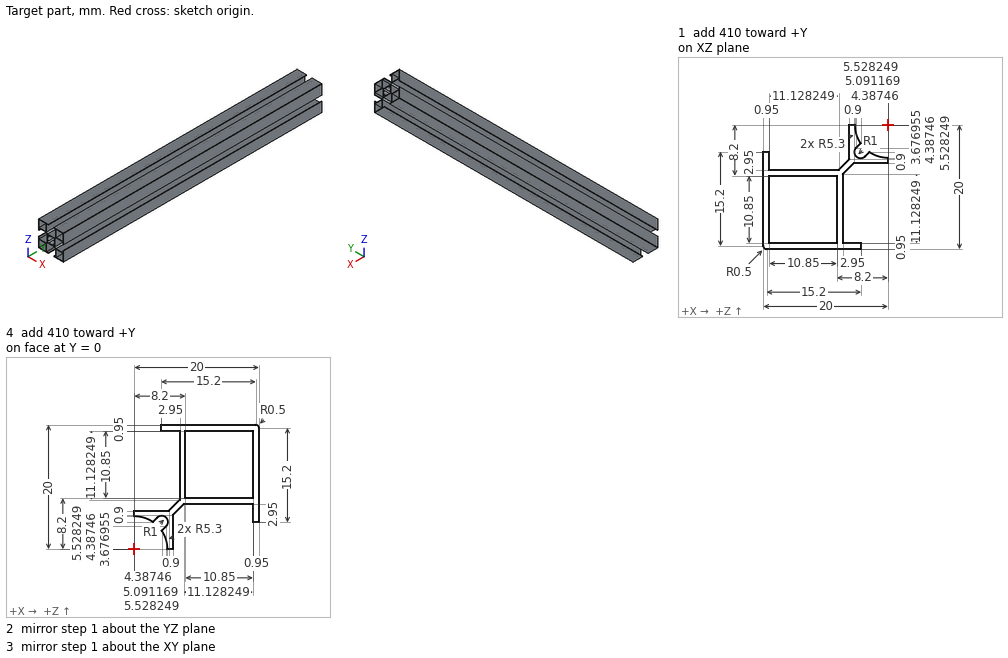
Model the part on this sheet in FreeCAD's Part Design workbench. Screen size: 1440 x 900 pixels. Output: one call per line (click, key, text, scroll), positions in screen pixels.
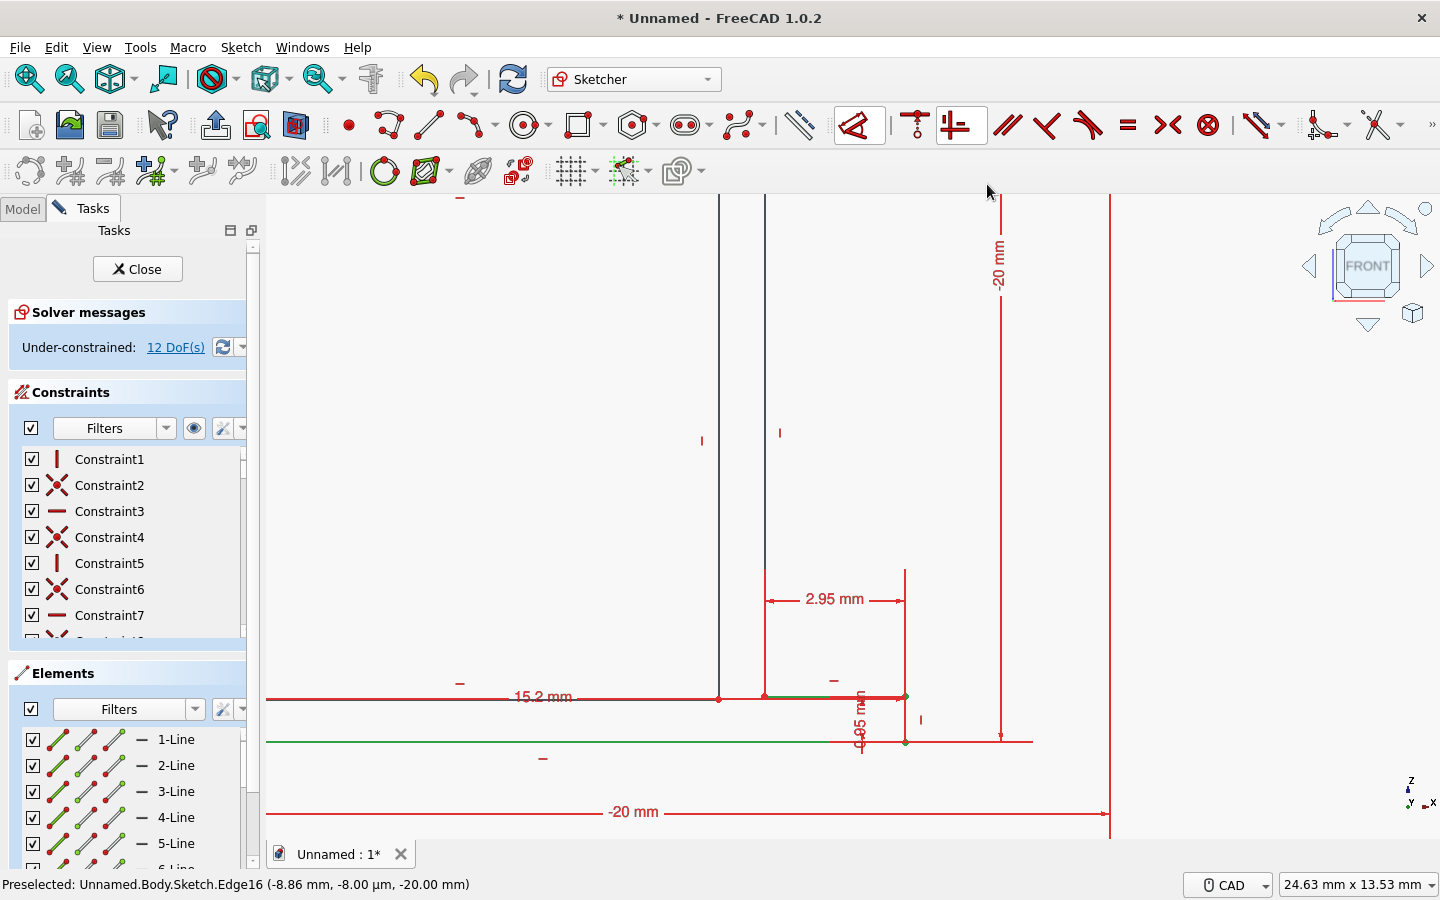
scroll(908, 721, down, 4)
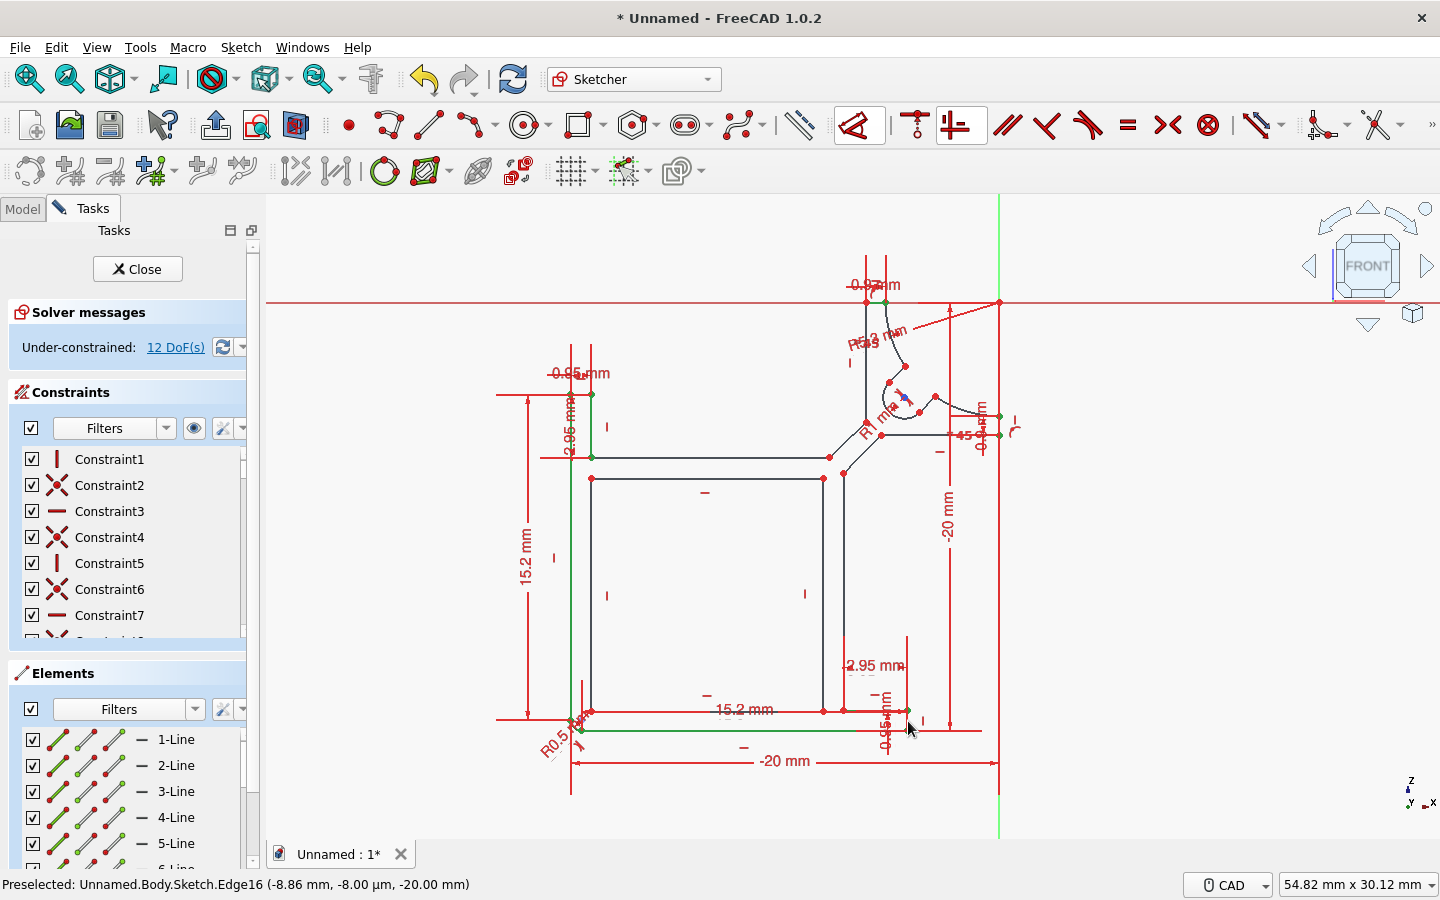
click(591, 479)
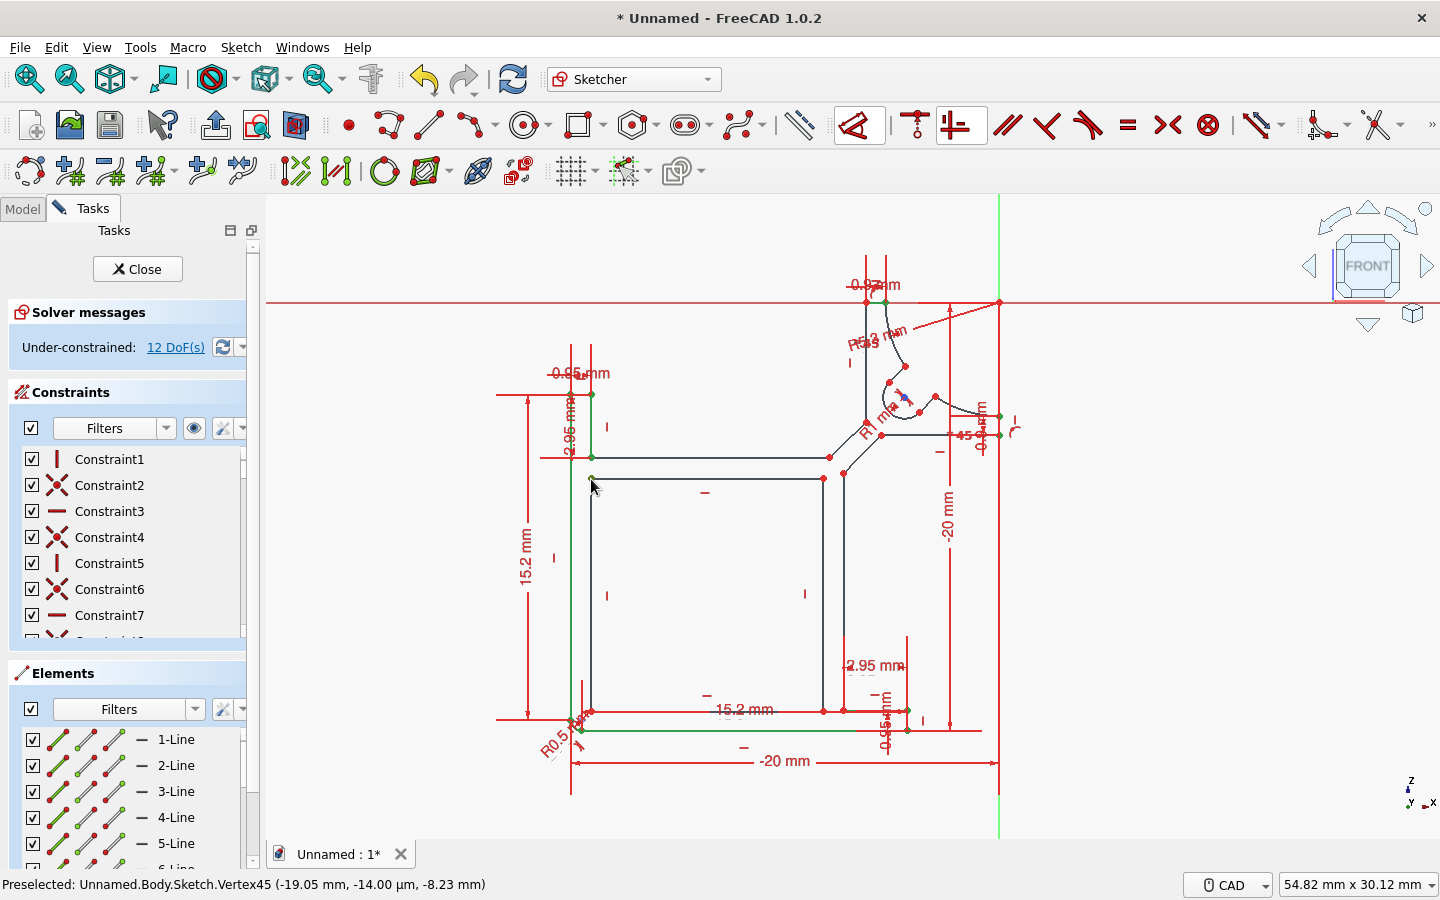
key(i)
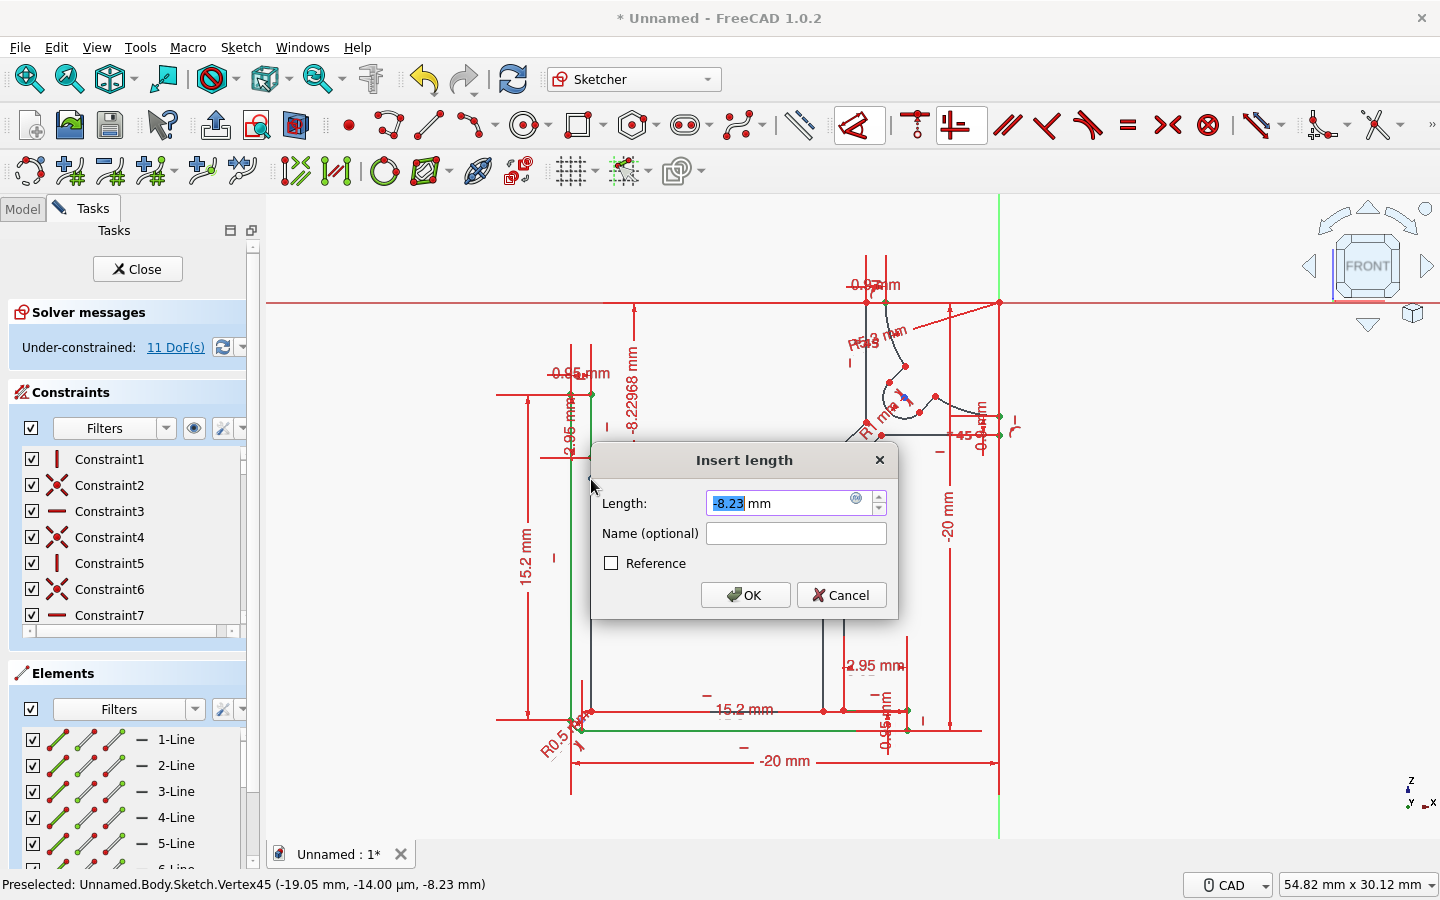
text(-8.2)
key(Return)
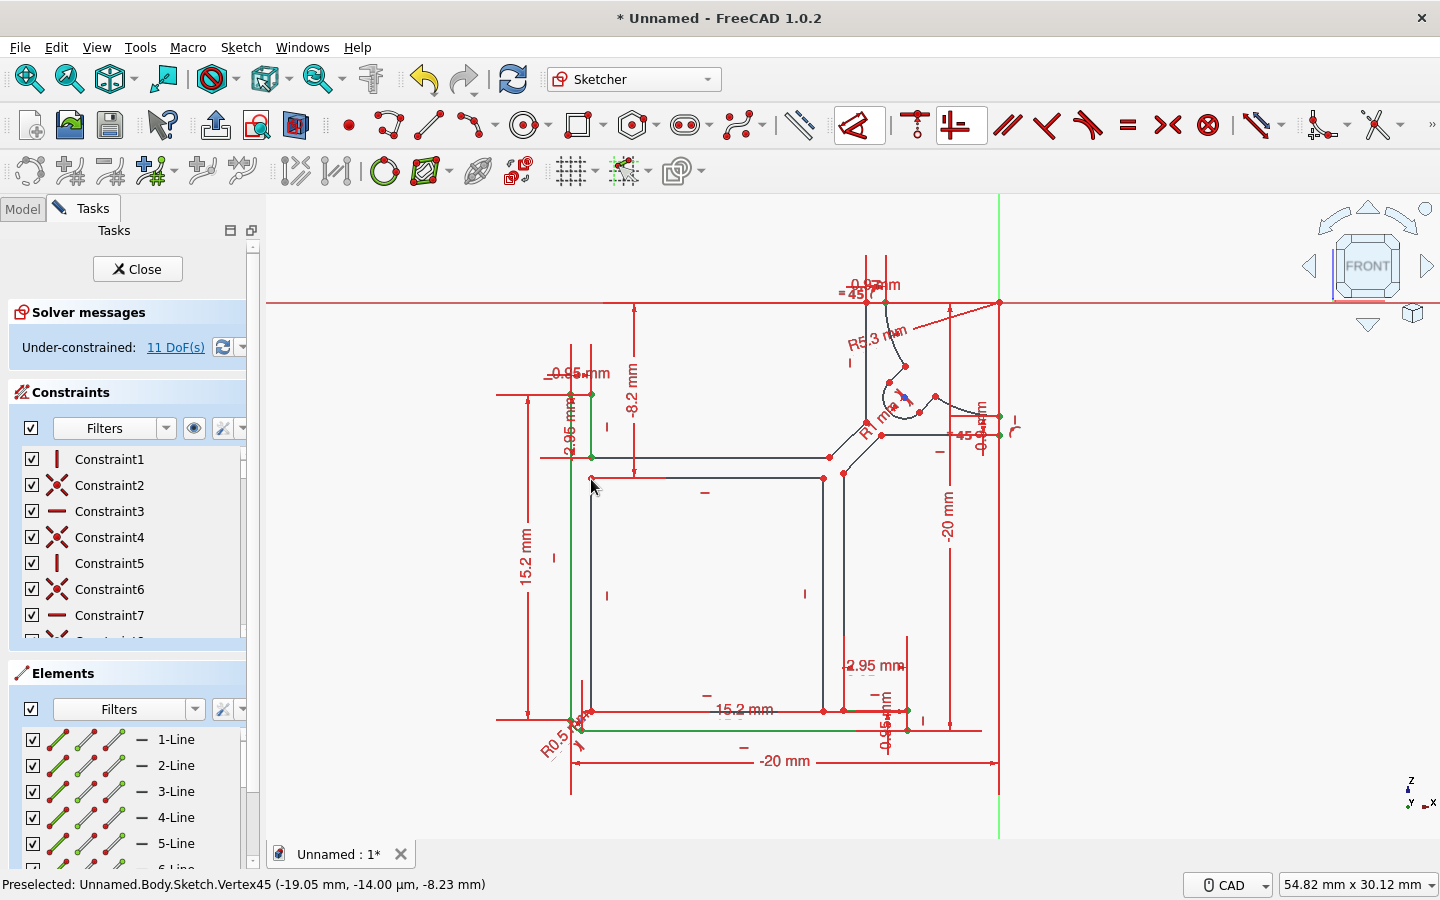
click(823, 712)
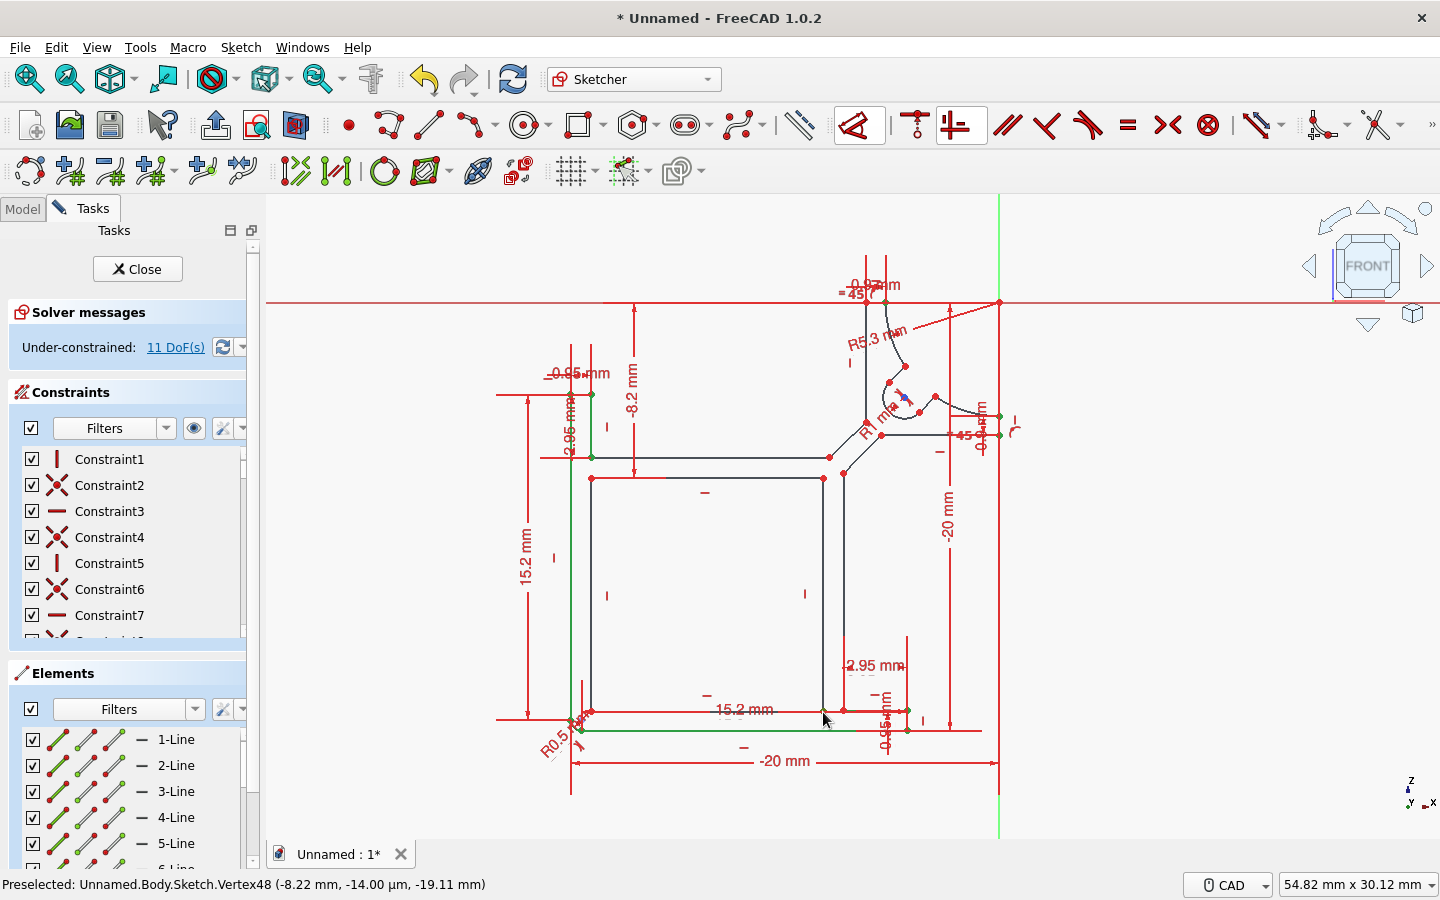
key(l)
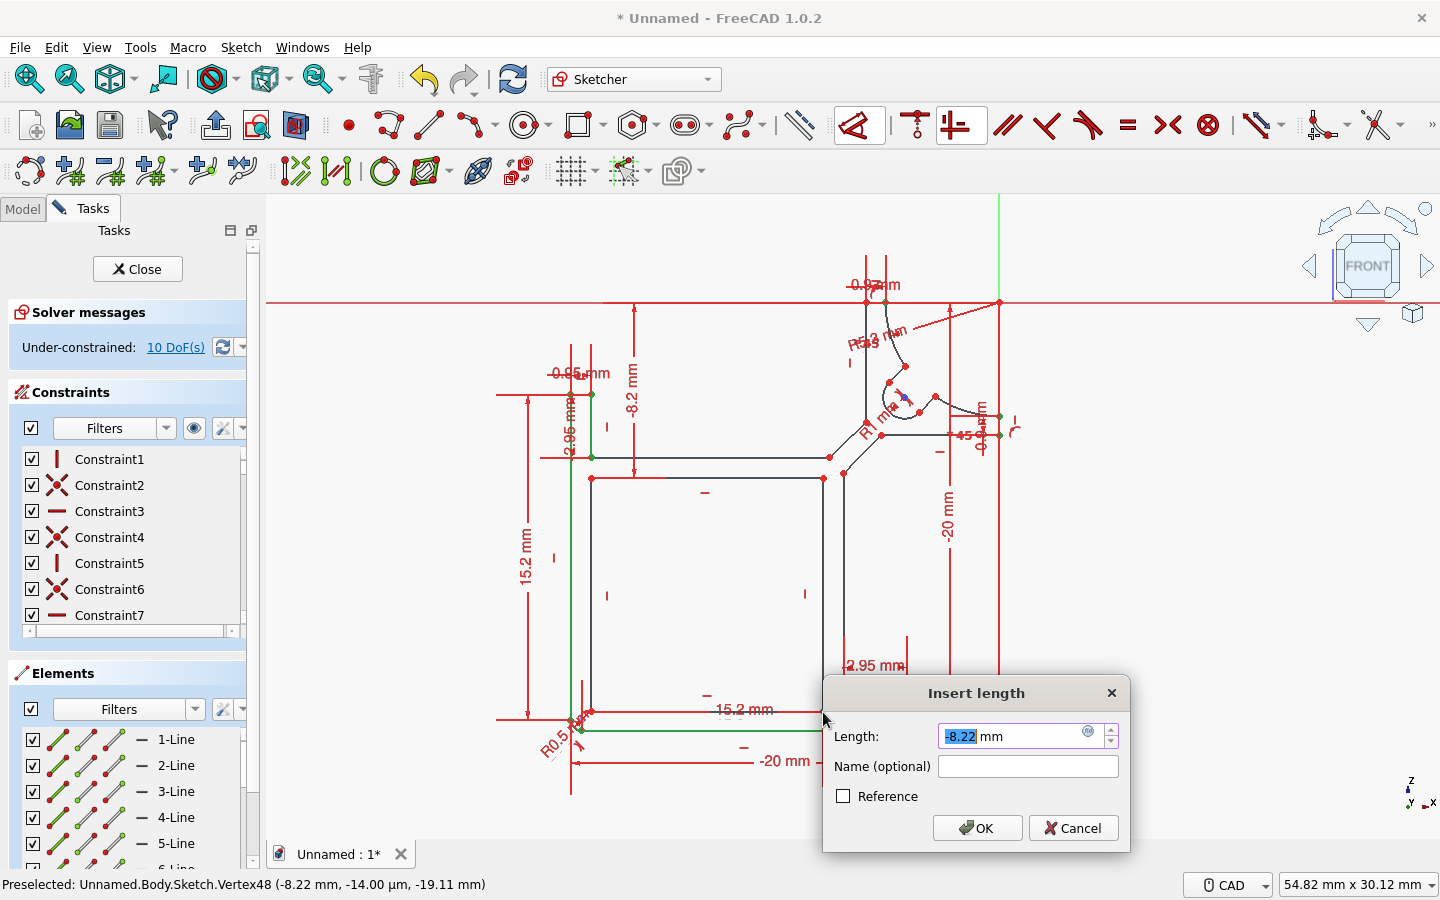
text(-8.2)
key(Return)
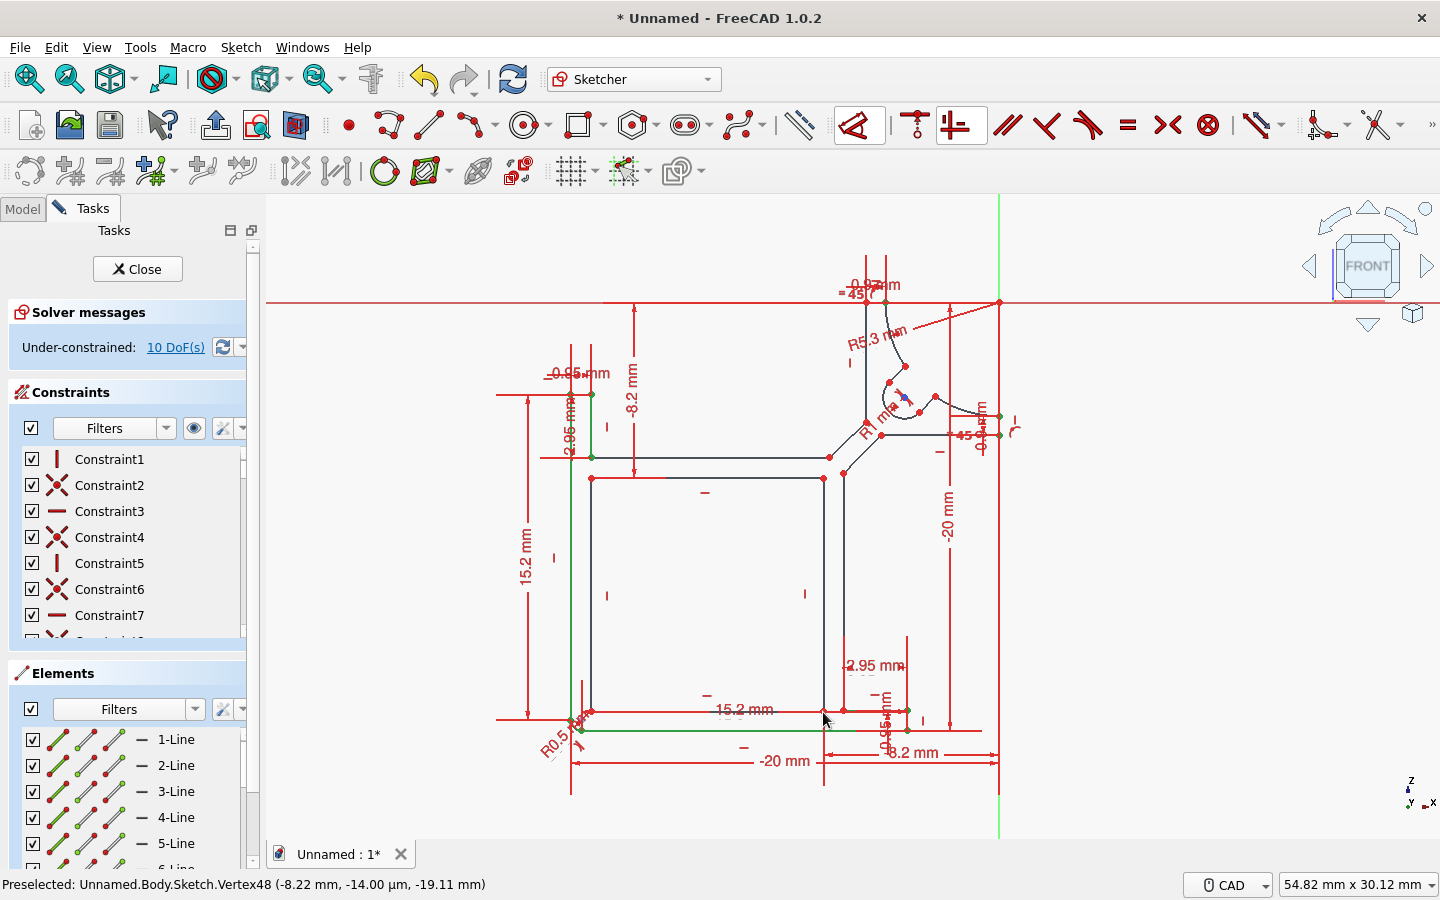
click(591, 548)